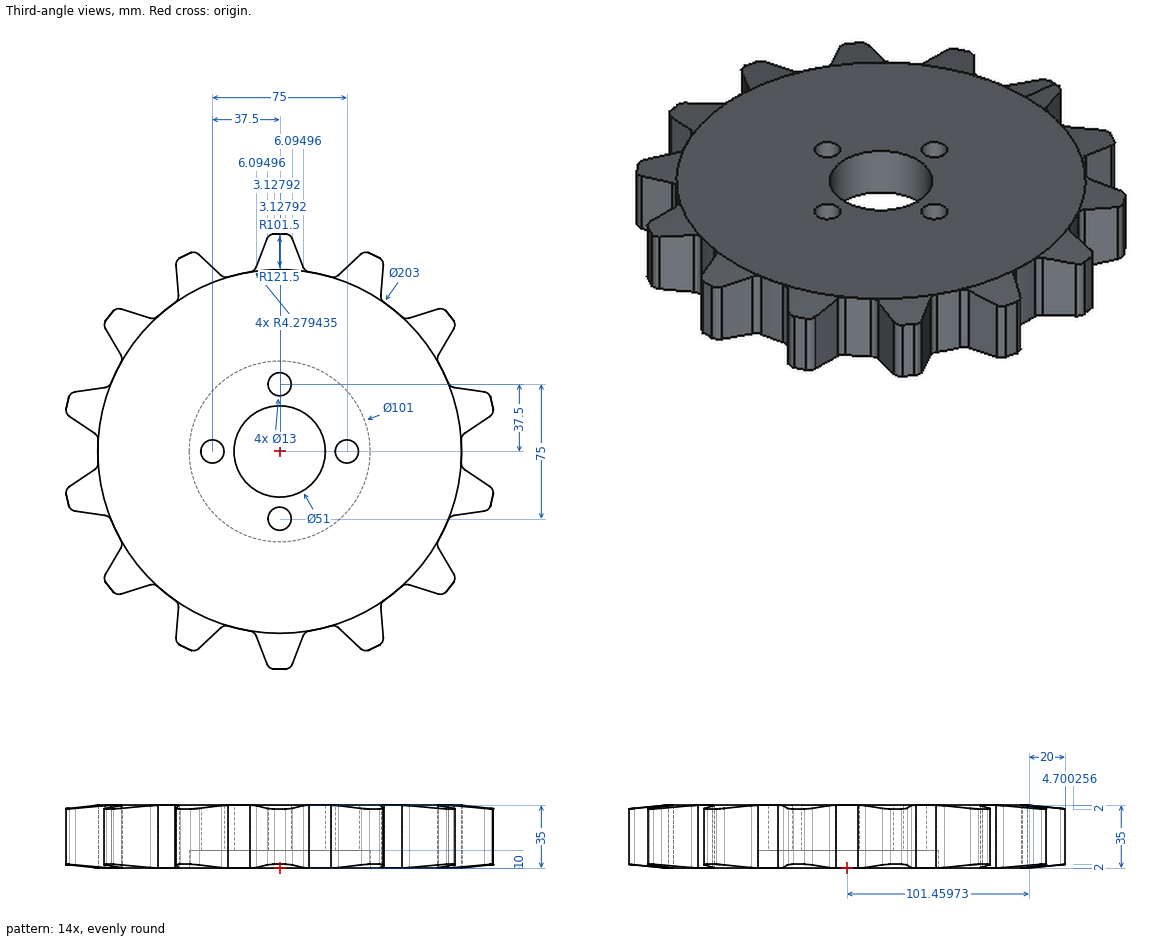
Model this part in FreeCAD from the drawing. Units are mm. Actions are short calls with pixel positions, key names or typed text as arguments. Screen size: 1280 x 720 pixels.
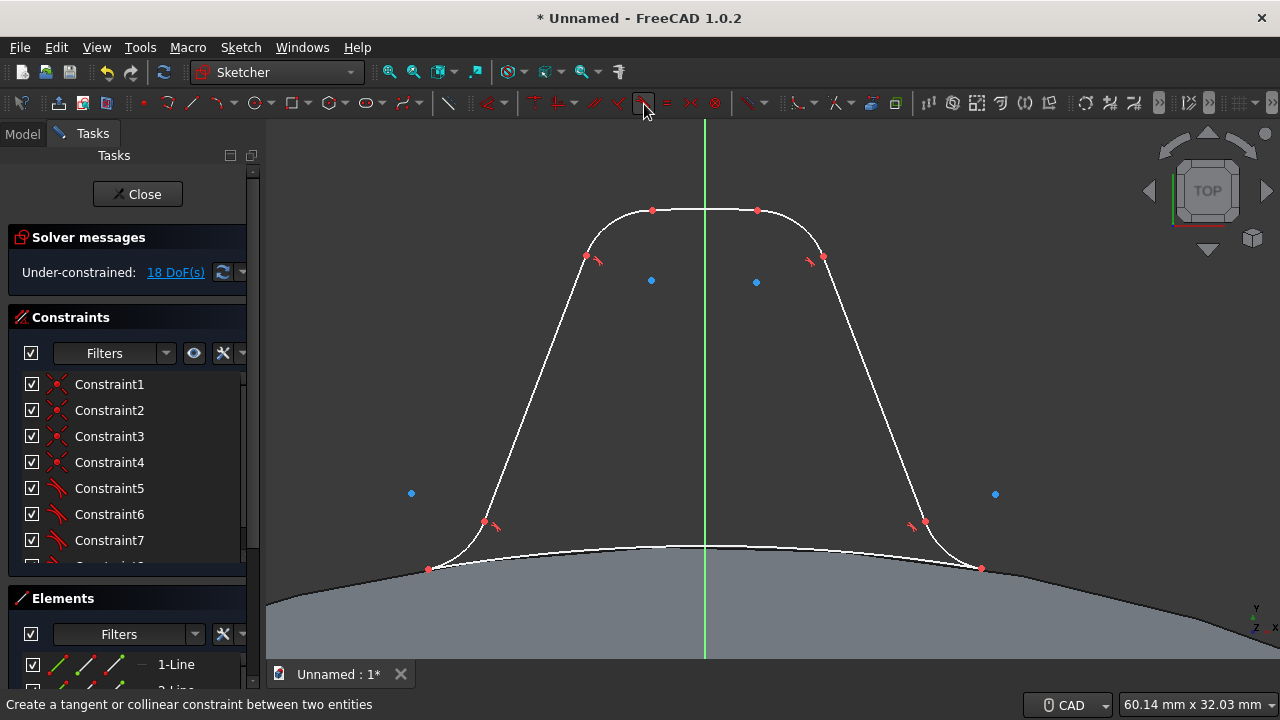
click(473, 541)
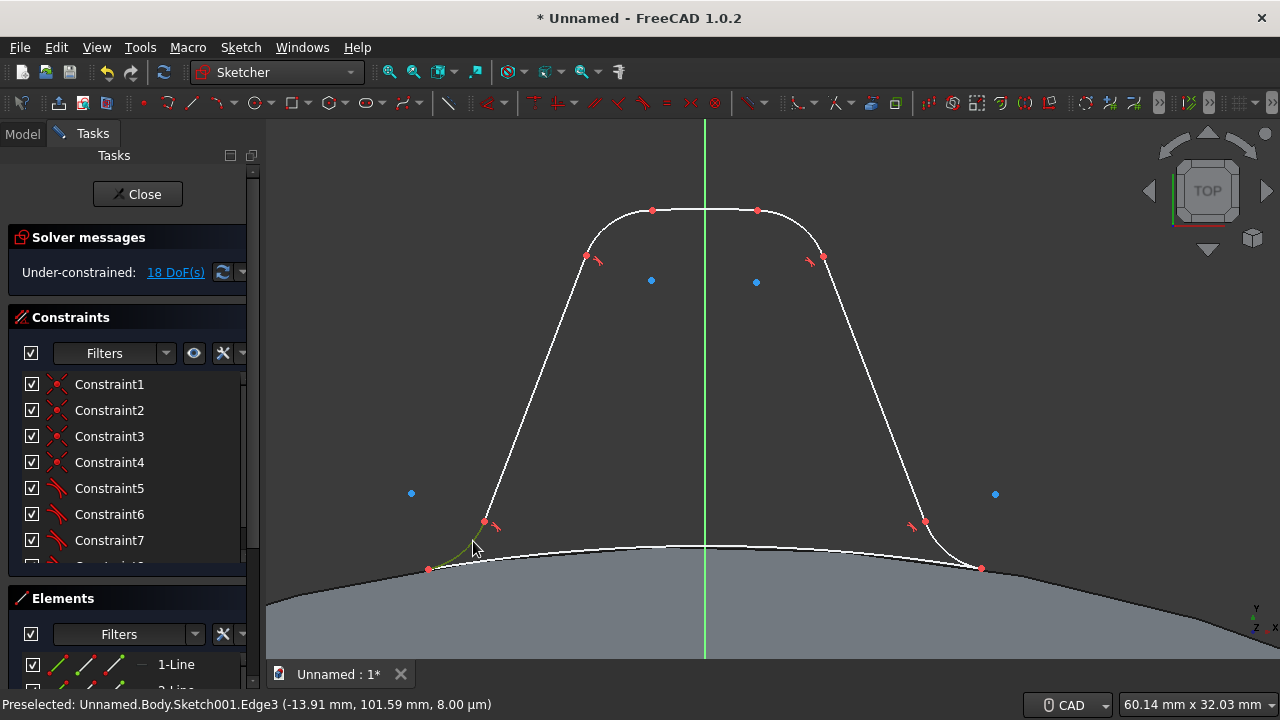
click(816, 550)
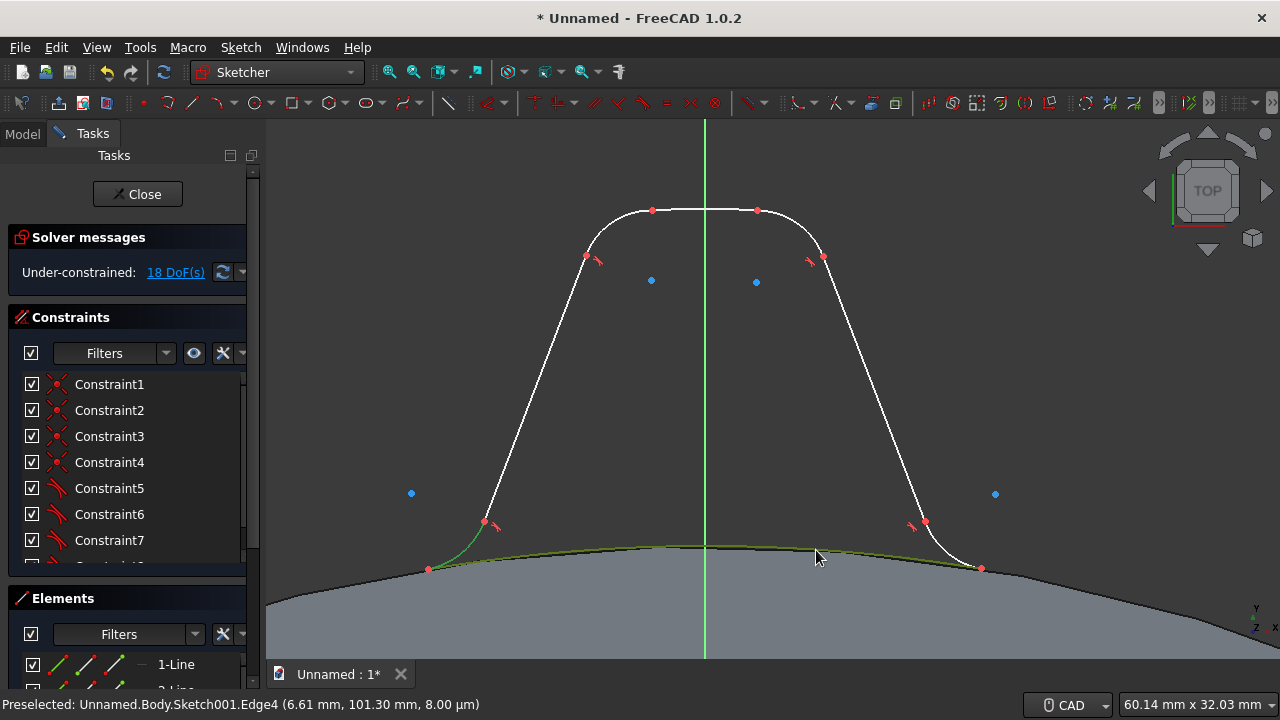
click(644, 104)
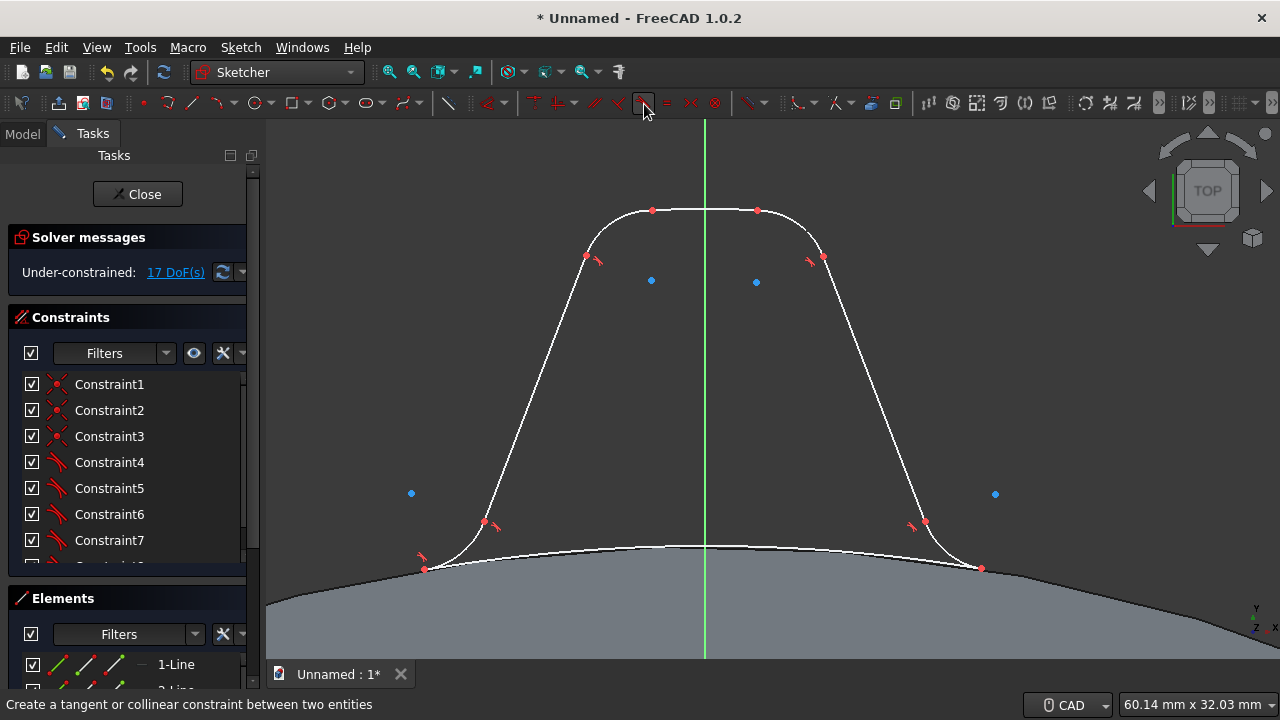
click(815, 550)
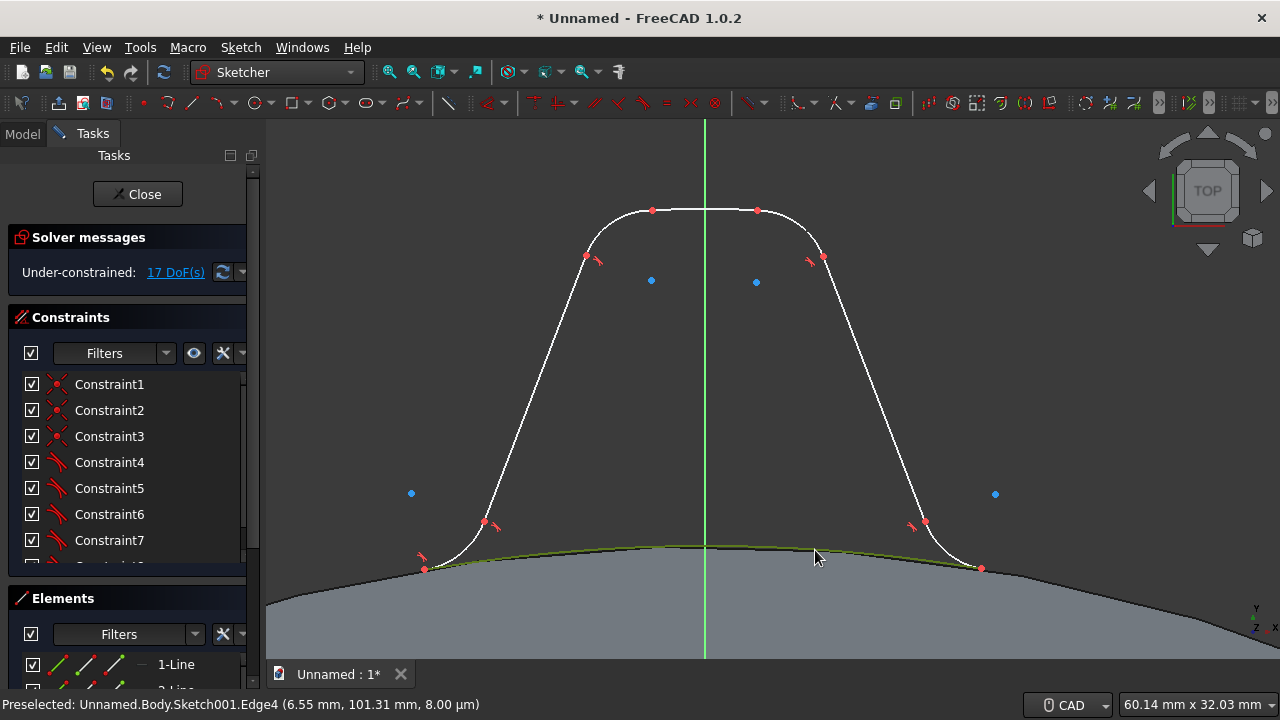
click(936, 542)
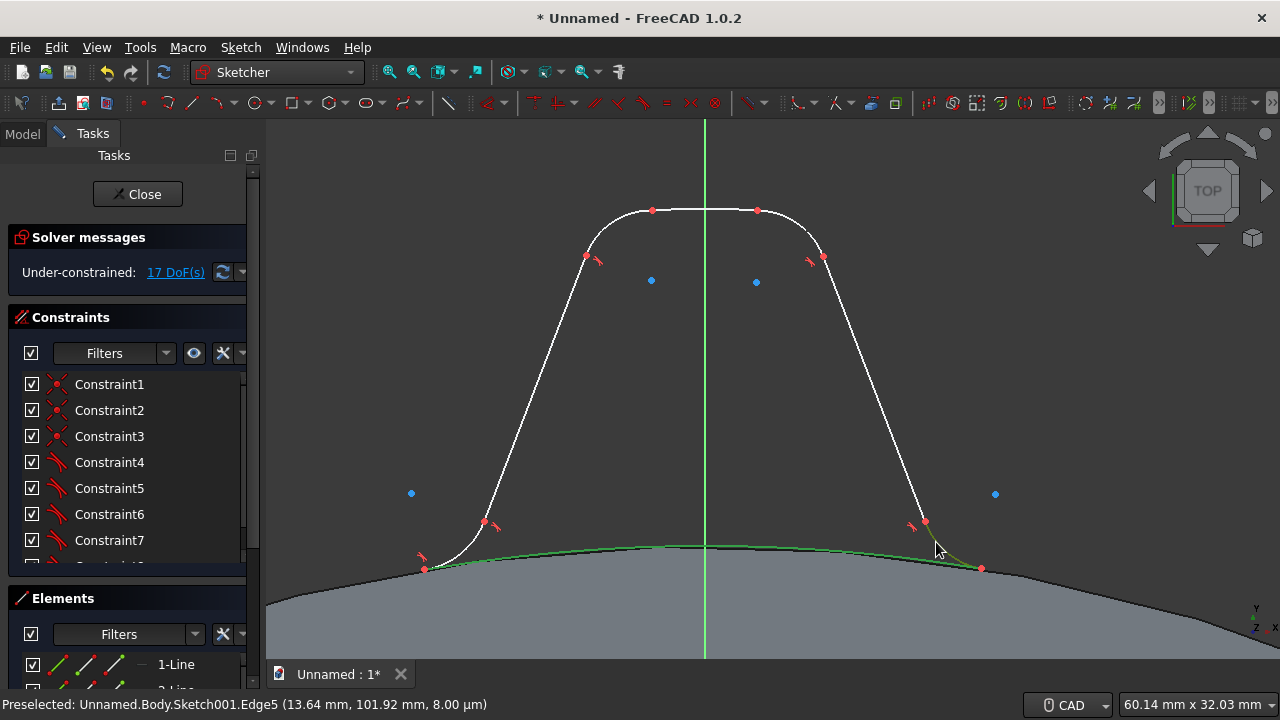
click(644, 104)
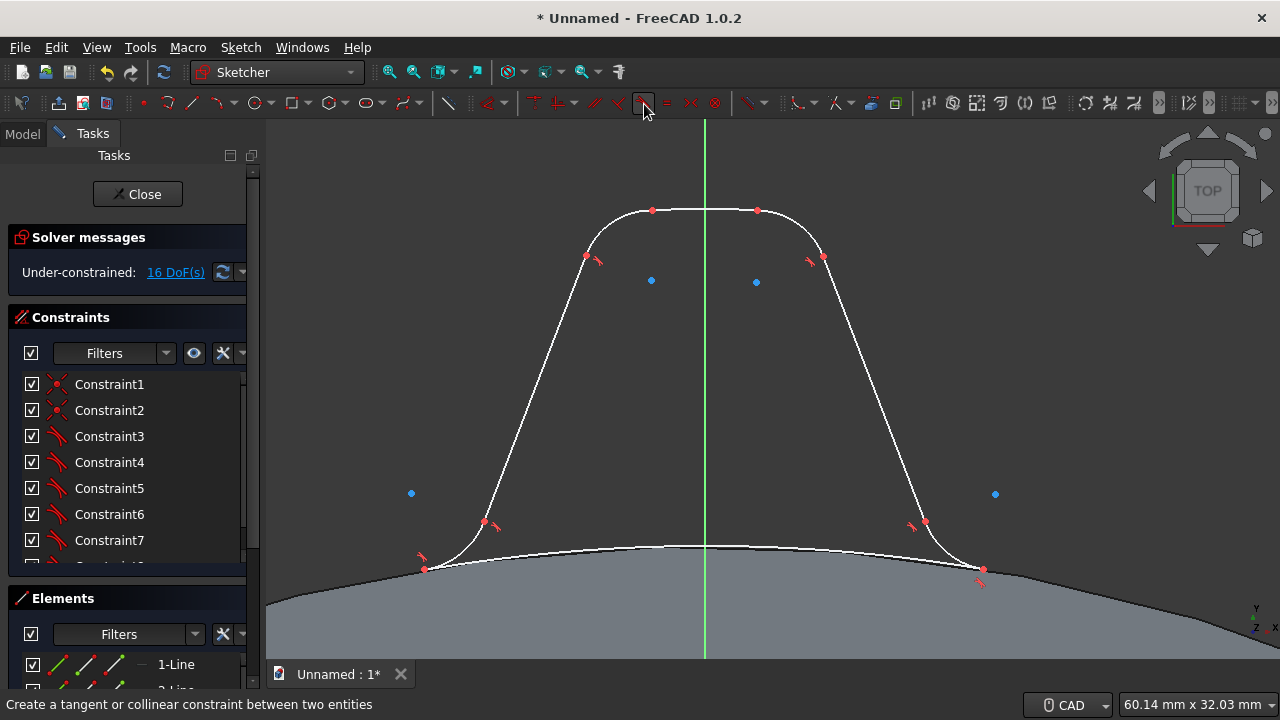
click(810, 235)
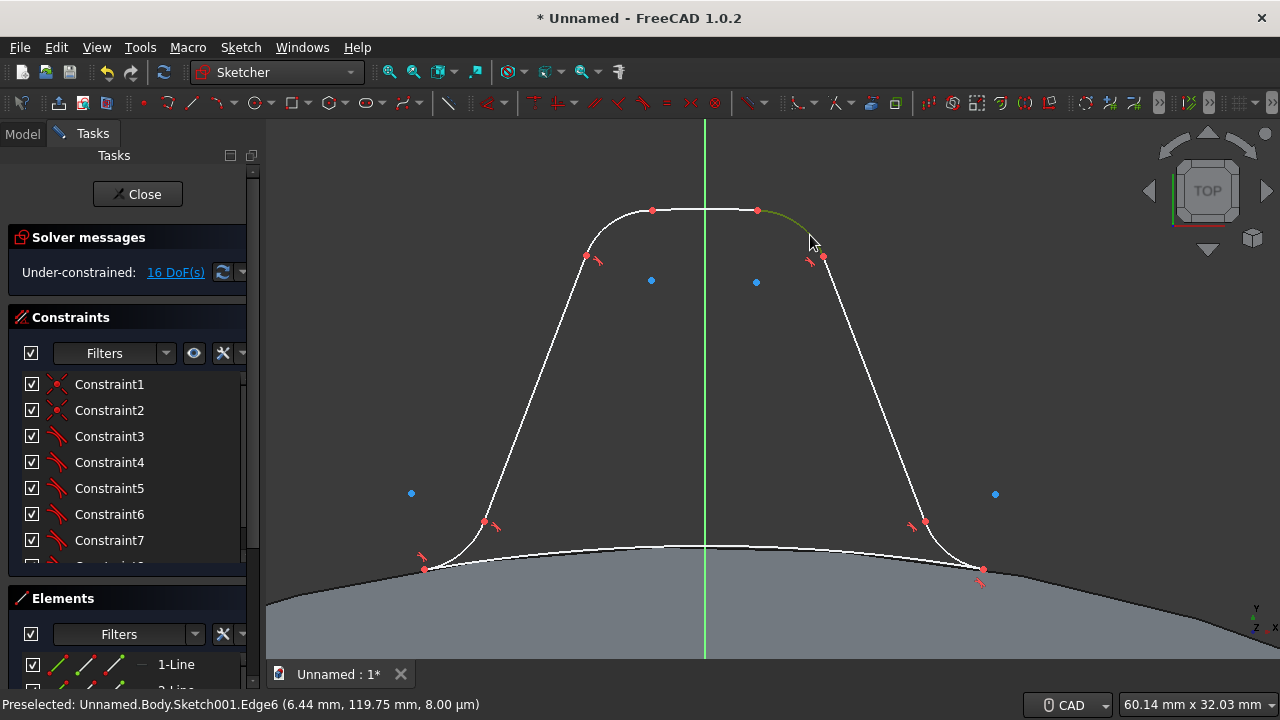
click(726, 209)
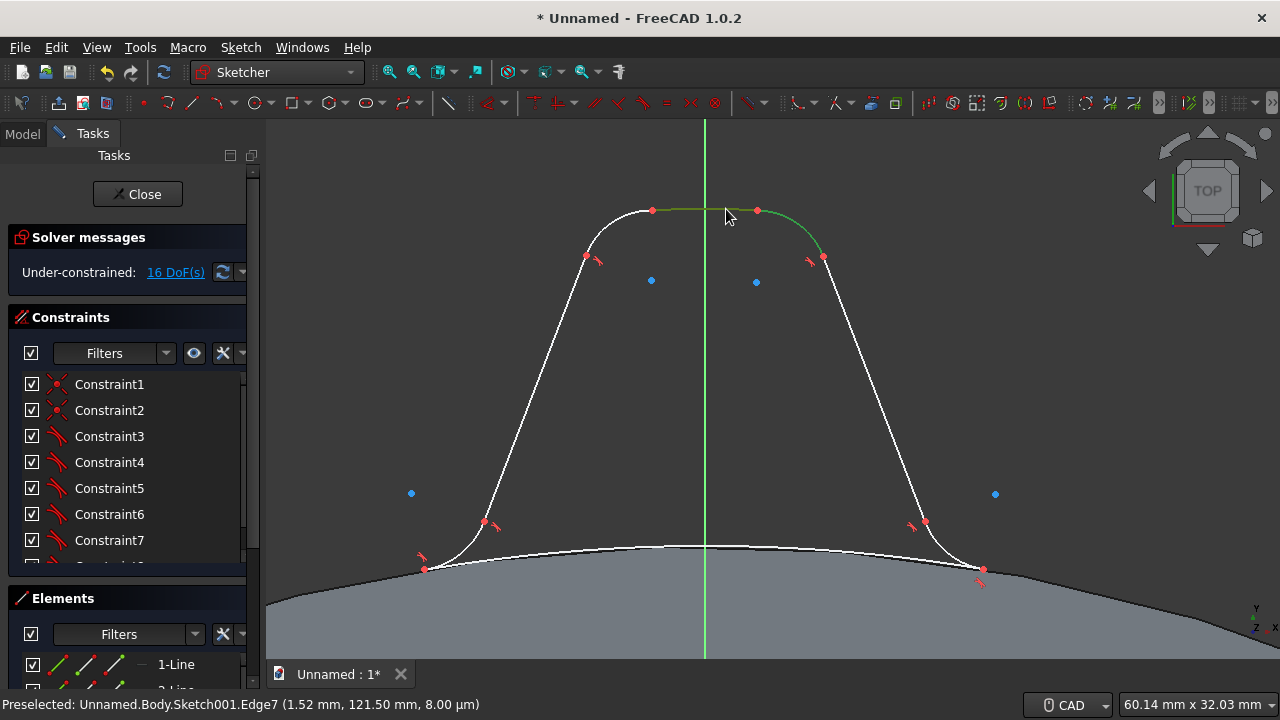
click(644, 104)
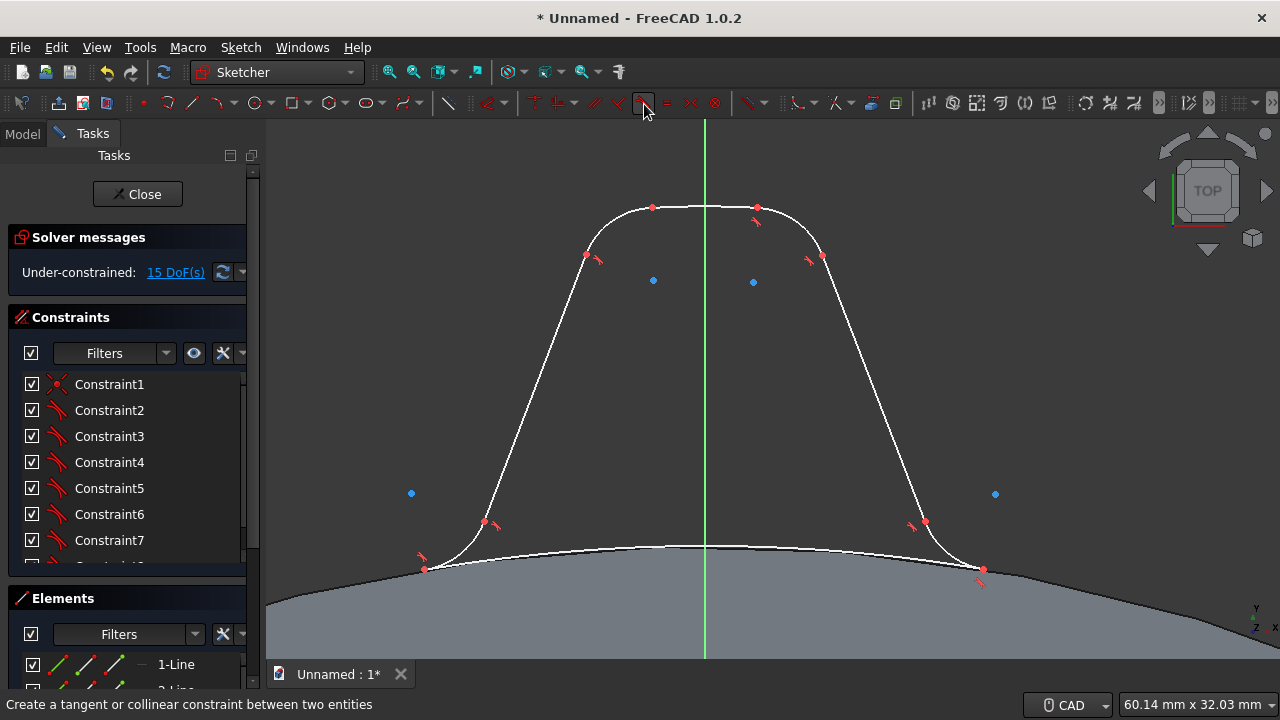
click(726, 207)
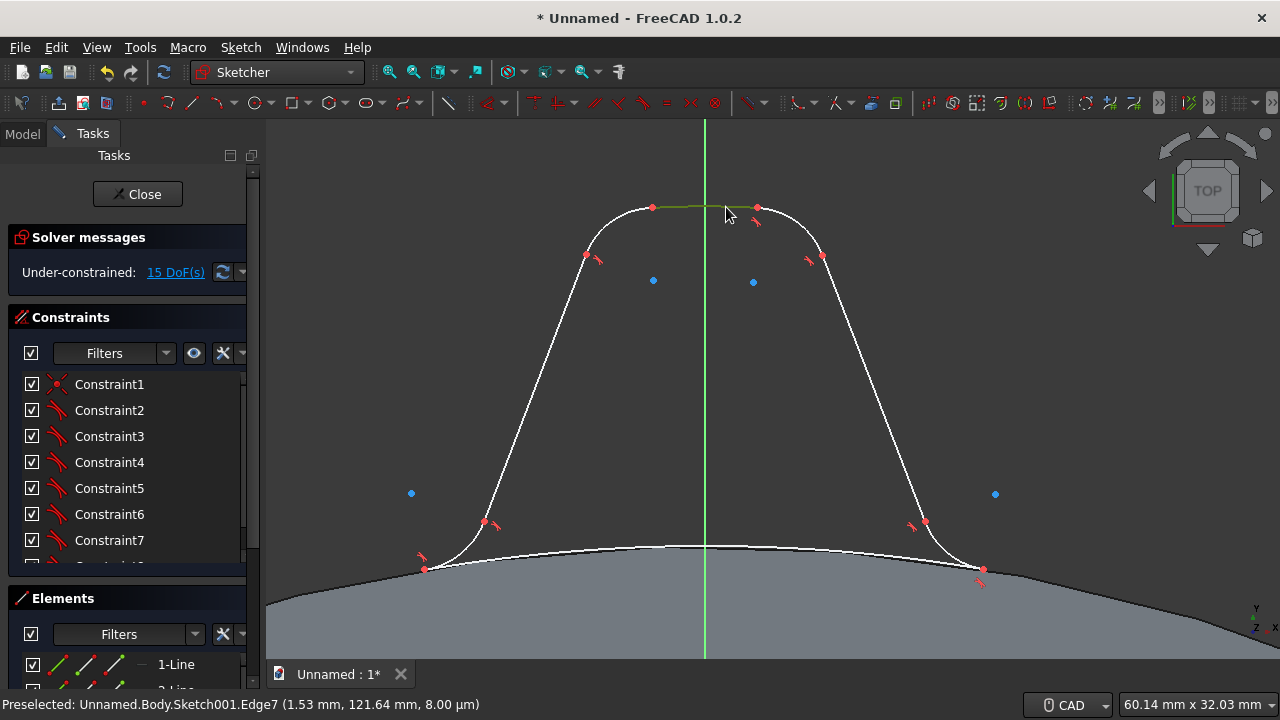
click(627, 213)